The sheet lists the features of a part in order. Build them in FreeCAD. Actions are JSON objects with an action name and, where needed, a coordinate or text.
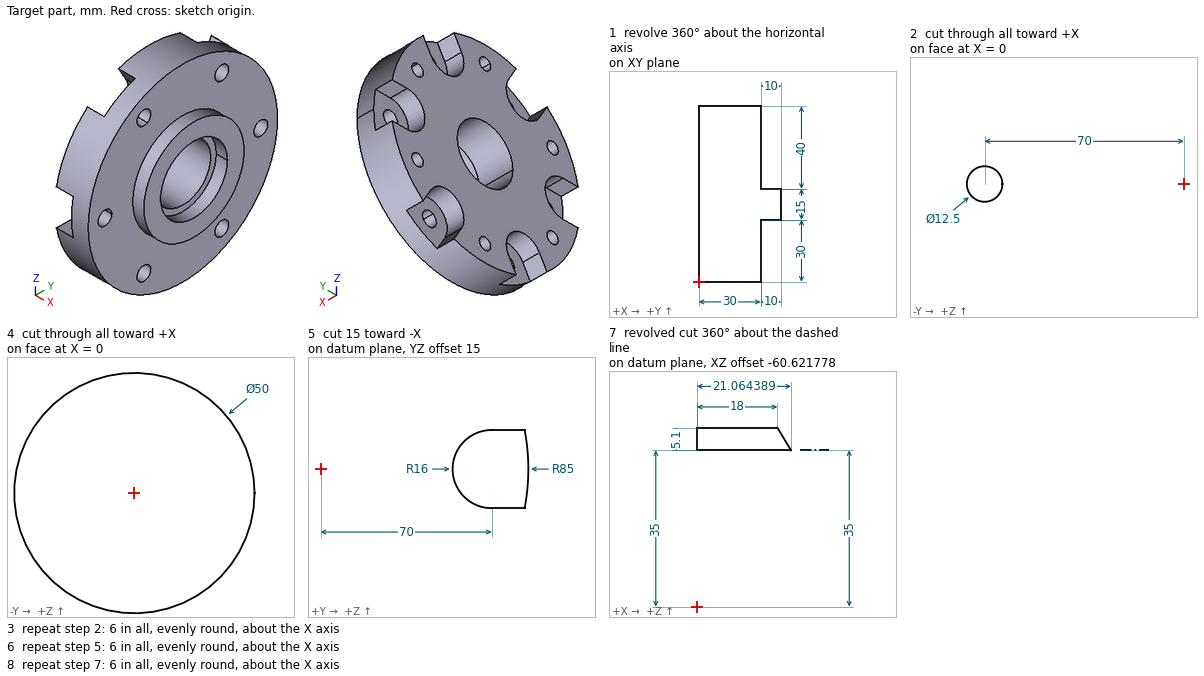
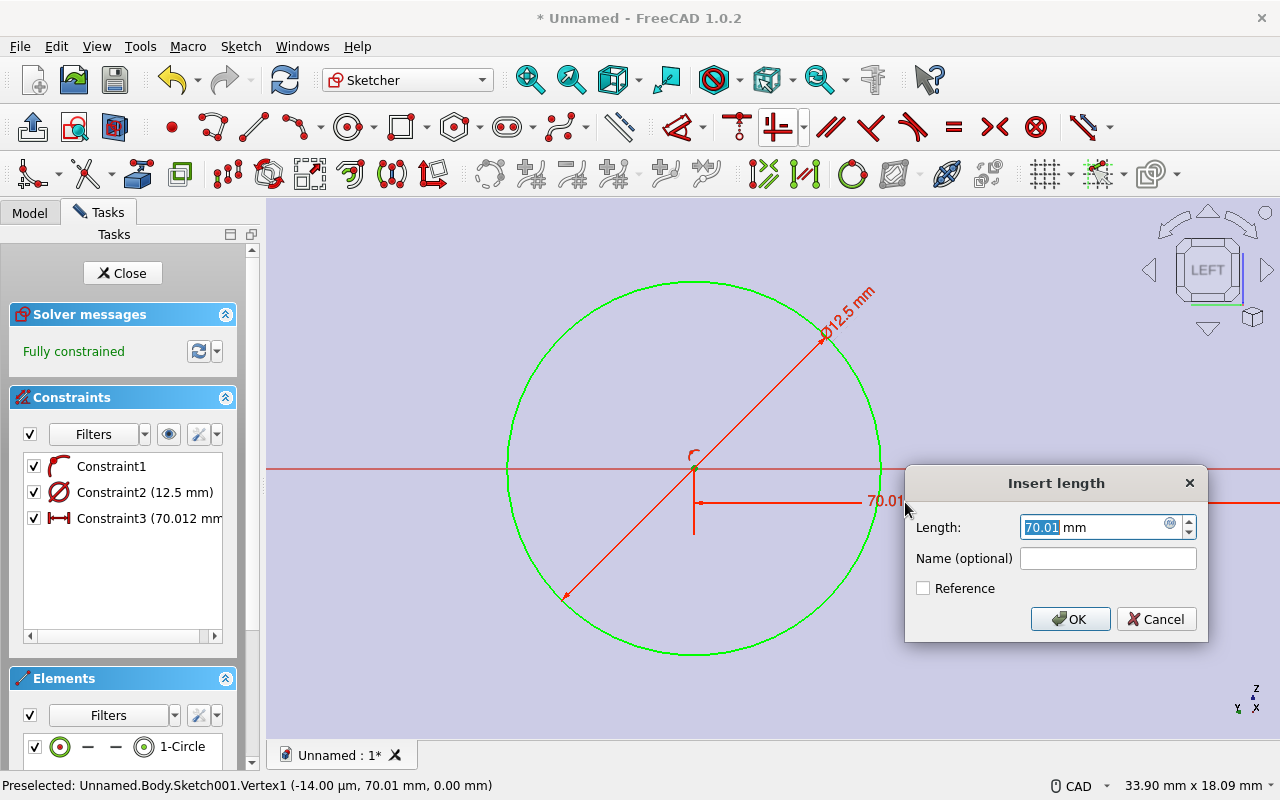
{"action": "type", "text": "70"}
{"action": "key", "text": "Return"}
{"action": "key", "text": "Escape"}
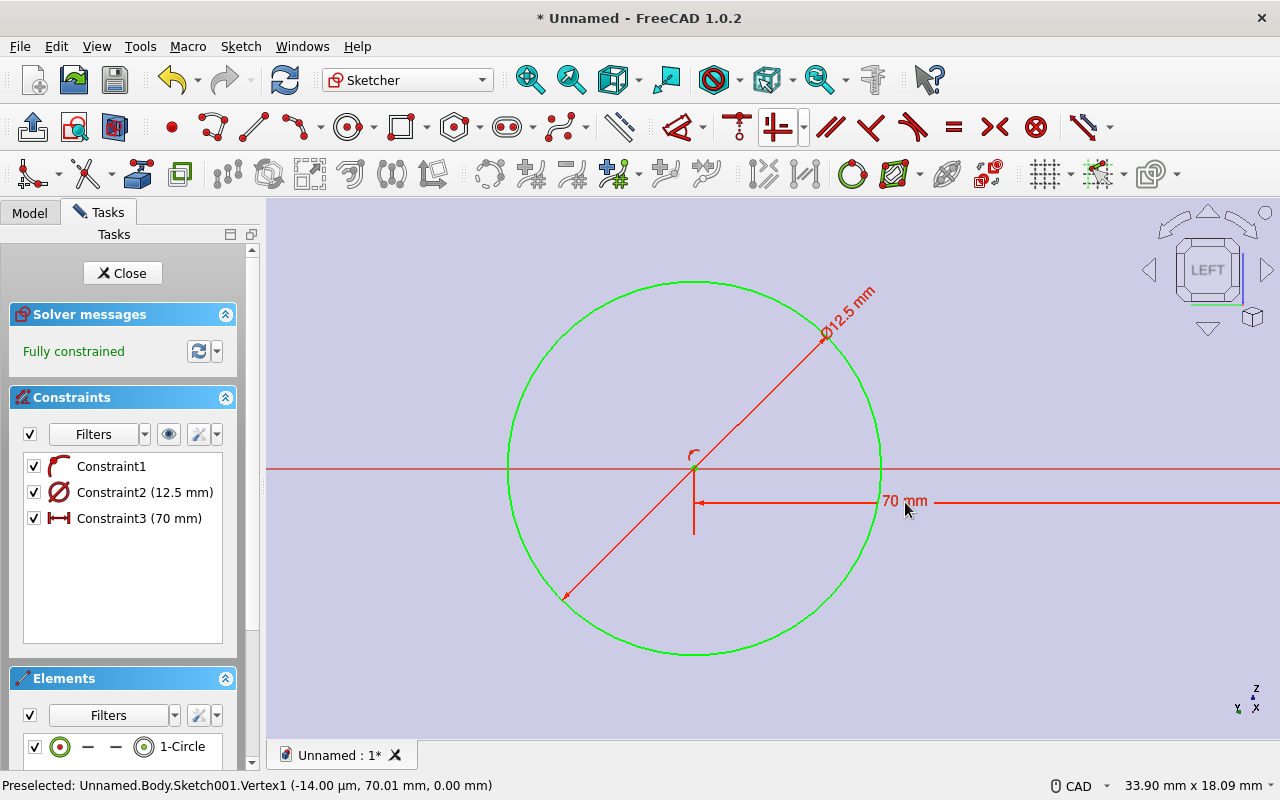
{"action": "left_click", "coordinate": [123, 273]}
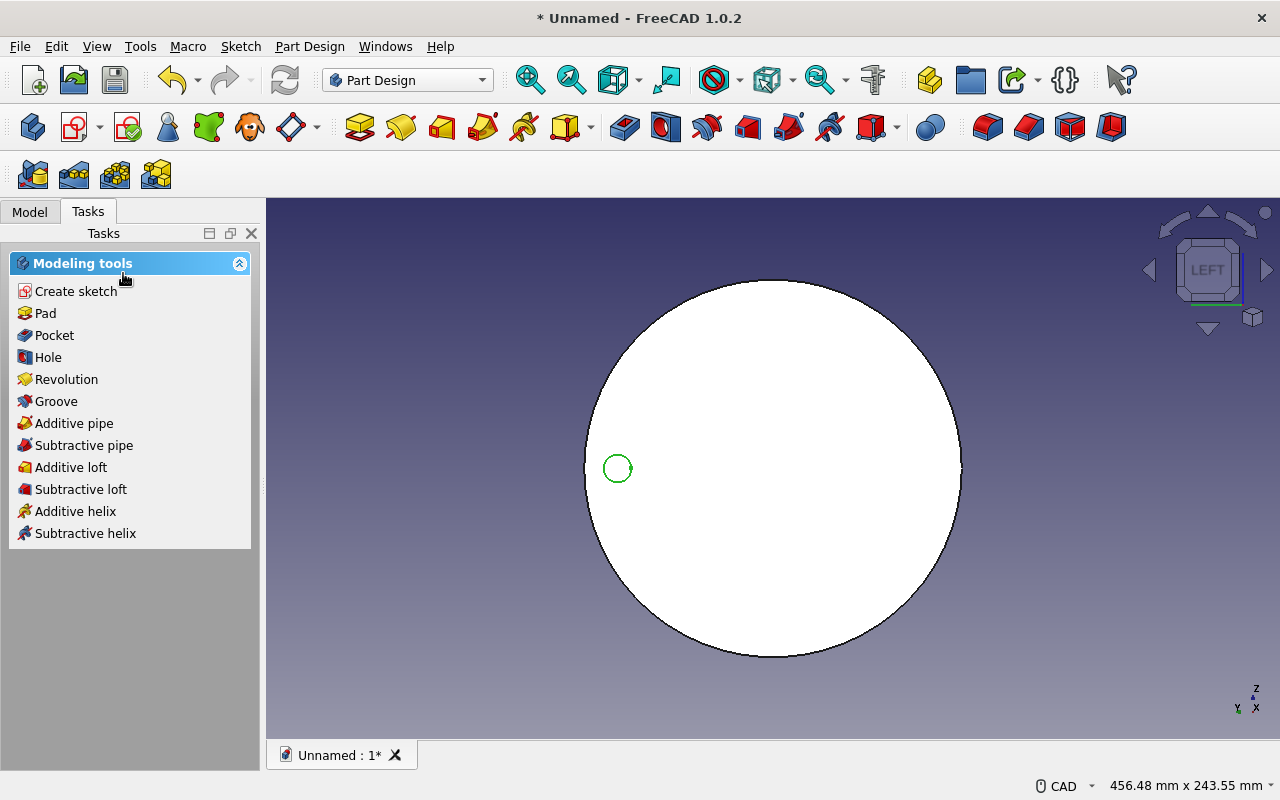
{"action": "left_click", "coordinate": [625, 128]}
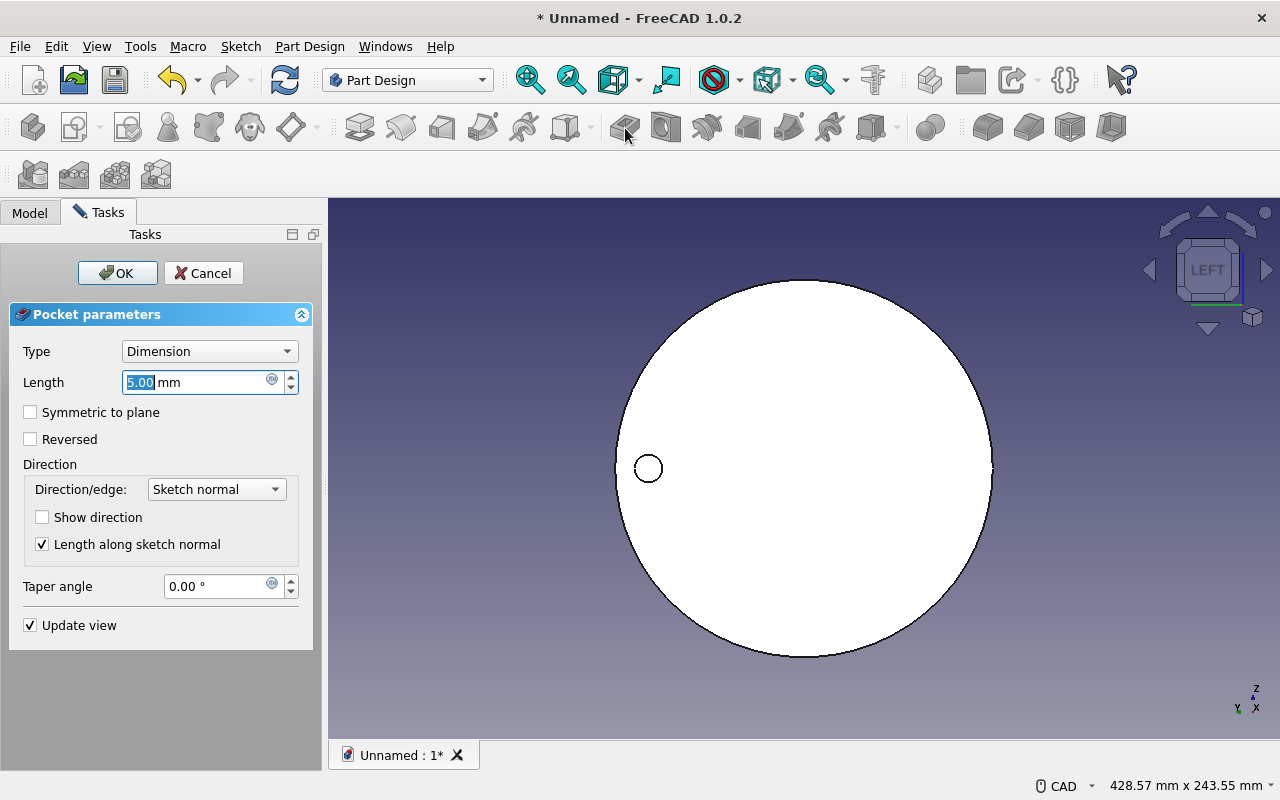
{"action": "left_click", "coordinate": [210, 352]}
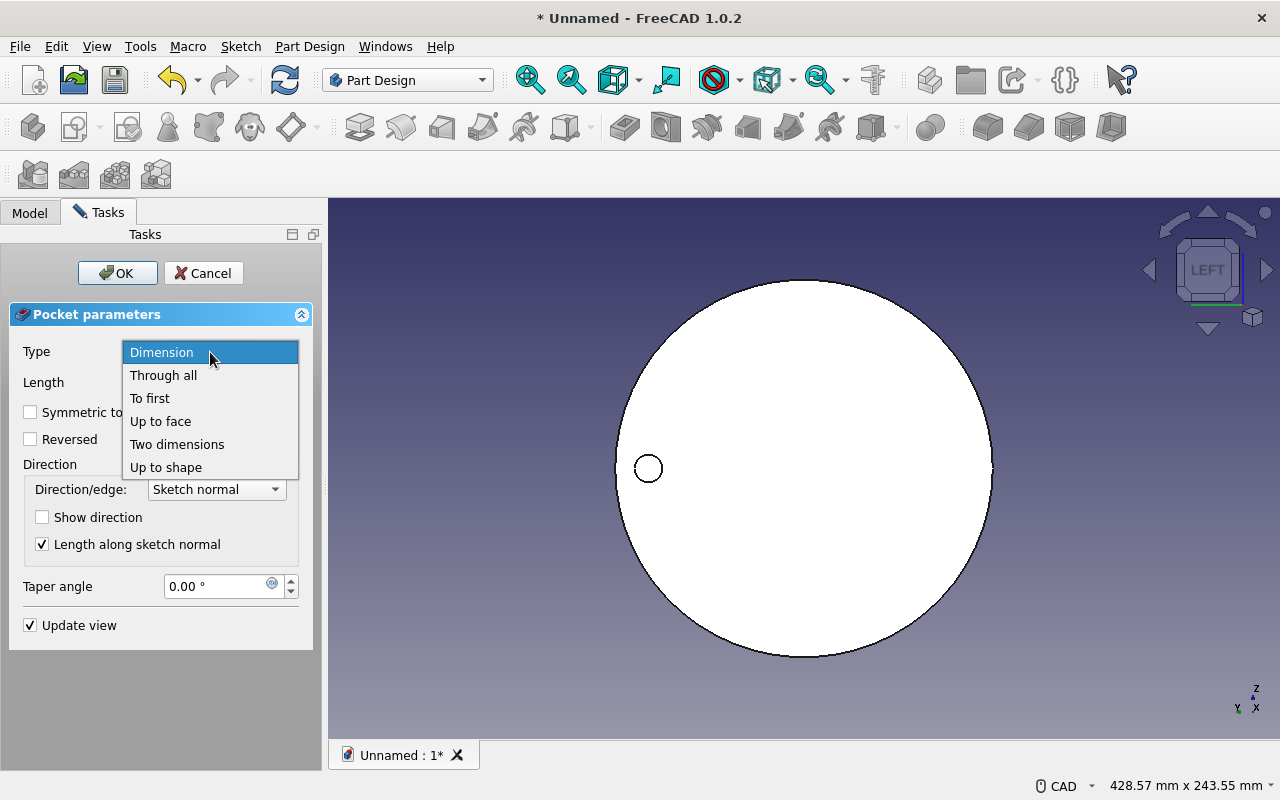
{"action": "left_click", "coordinate": [208, 376]}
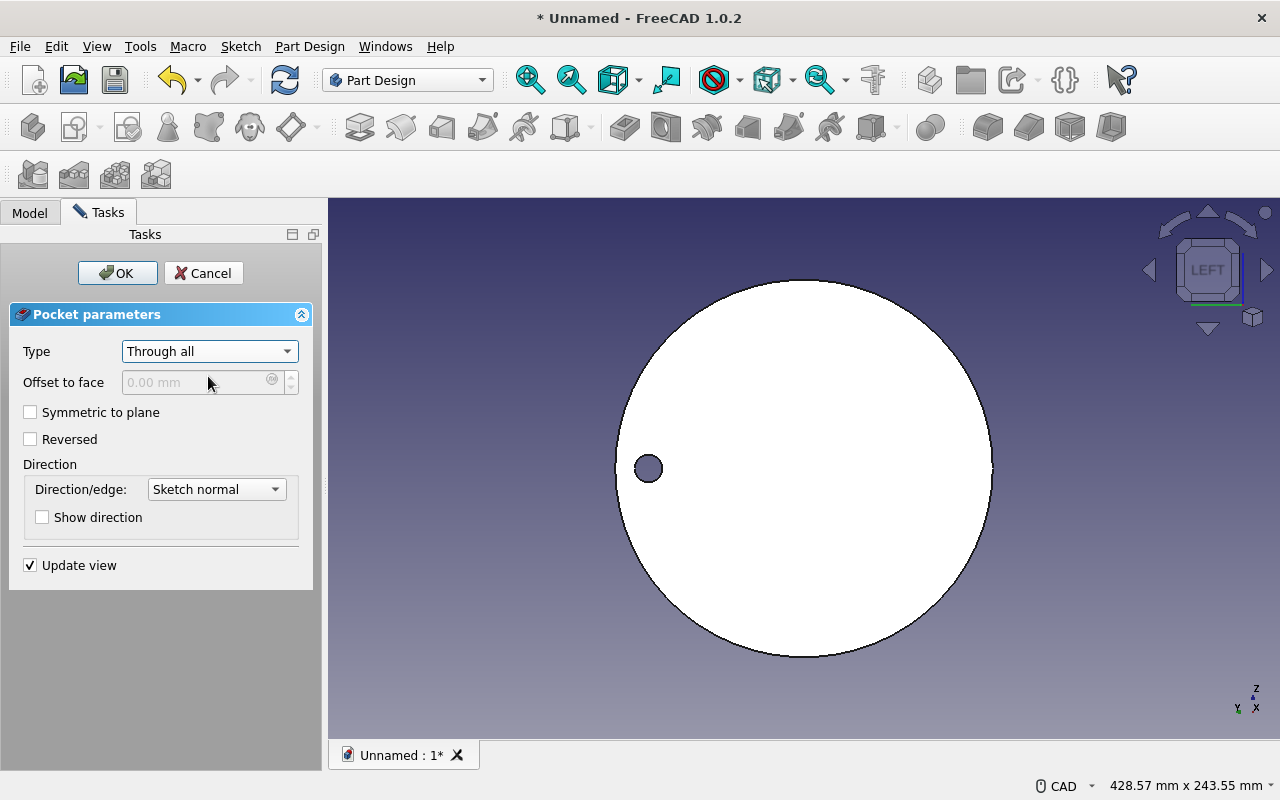
{"action": "left_click", "coordinate": [118, 273]}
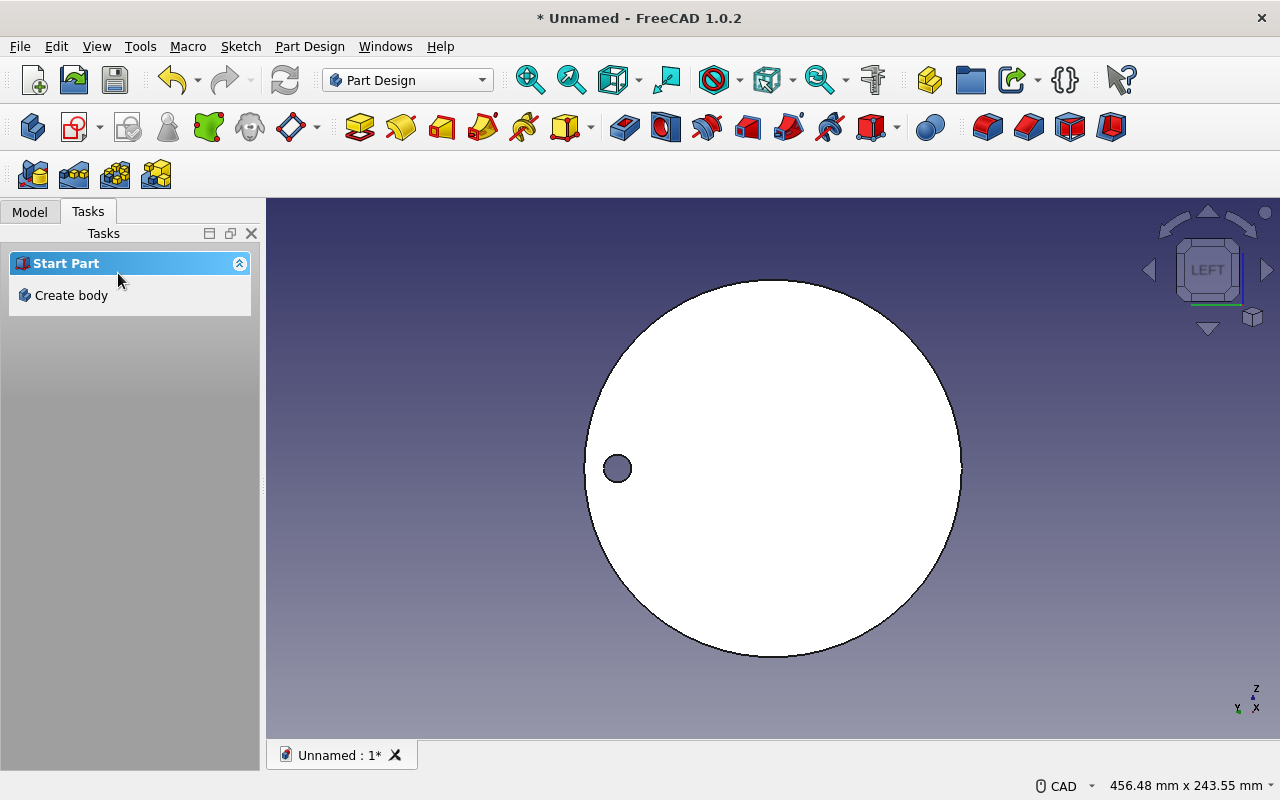
{"action": "left_click", "coordinate": [30, 212]}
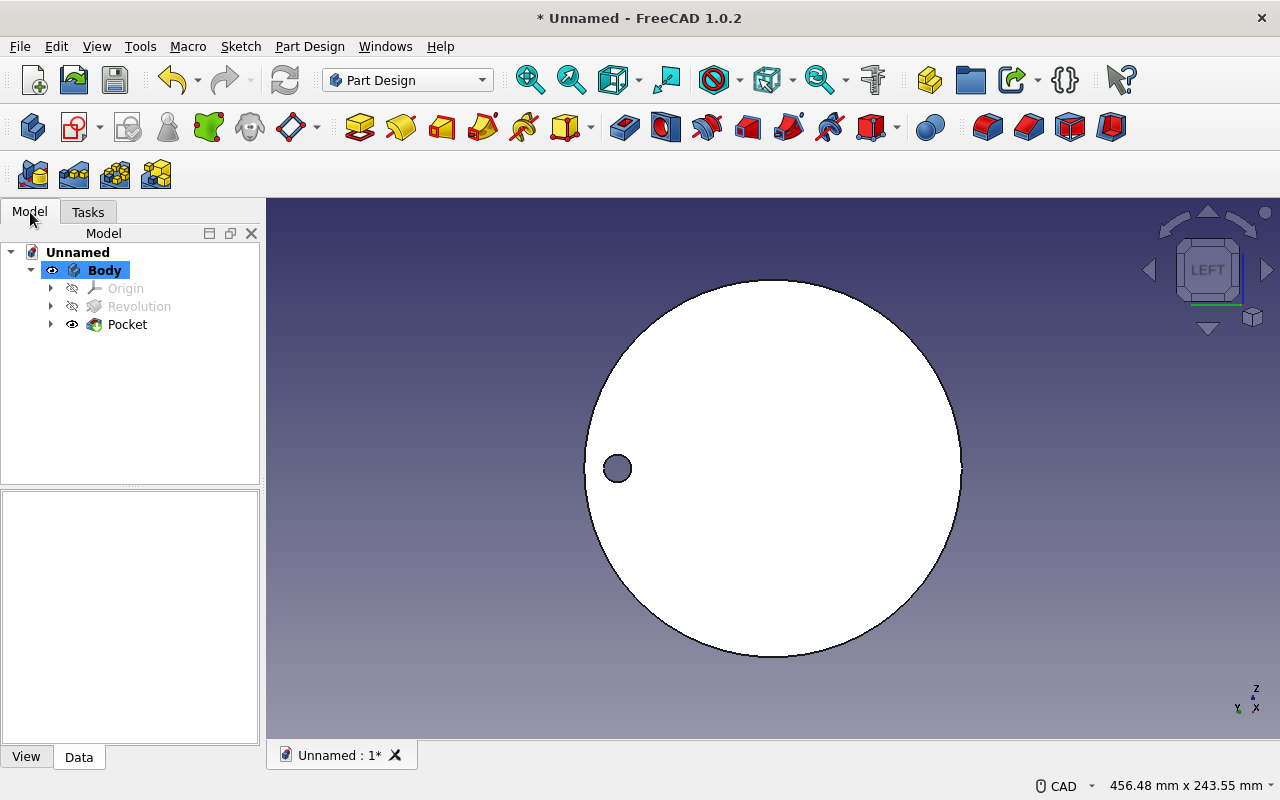
{"action": "left_click", "coordinate": [117, 324]}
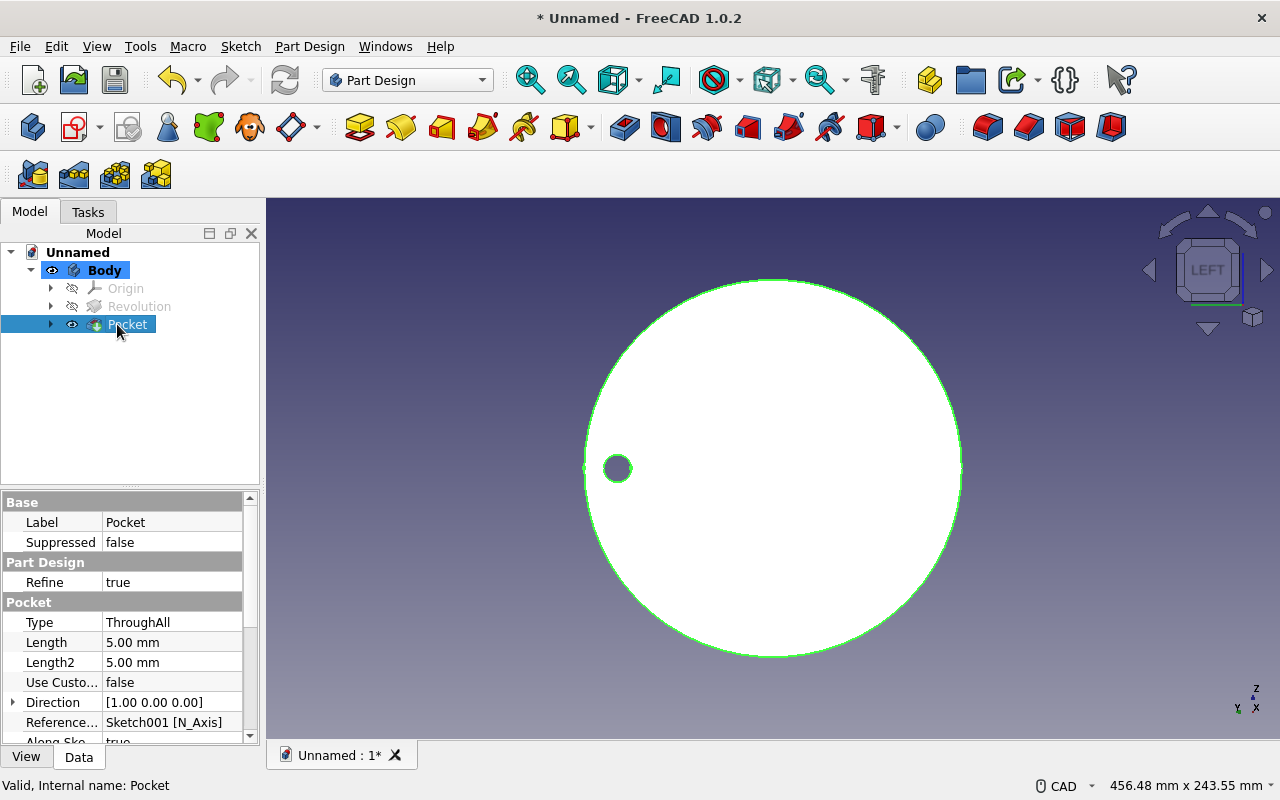
{"action": "left_click", "coordinate": [115, 174]}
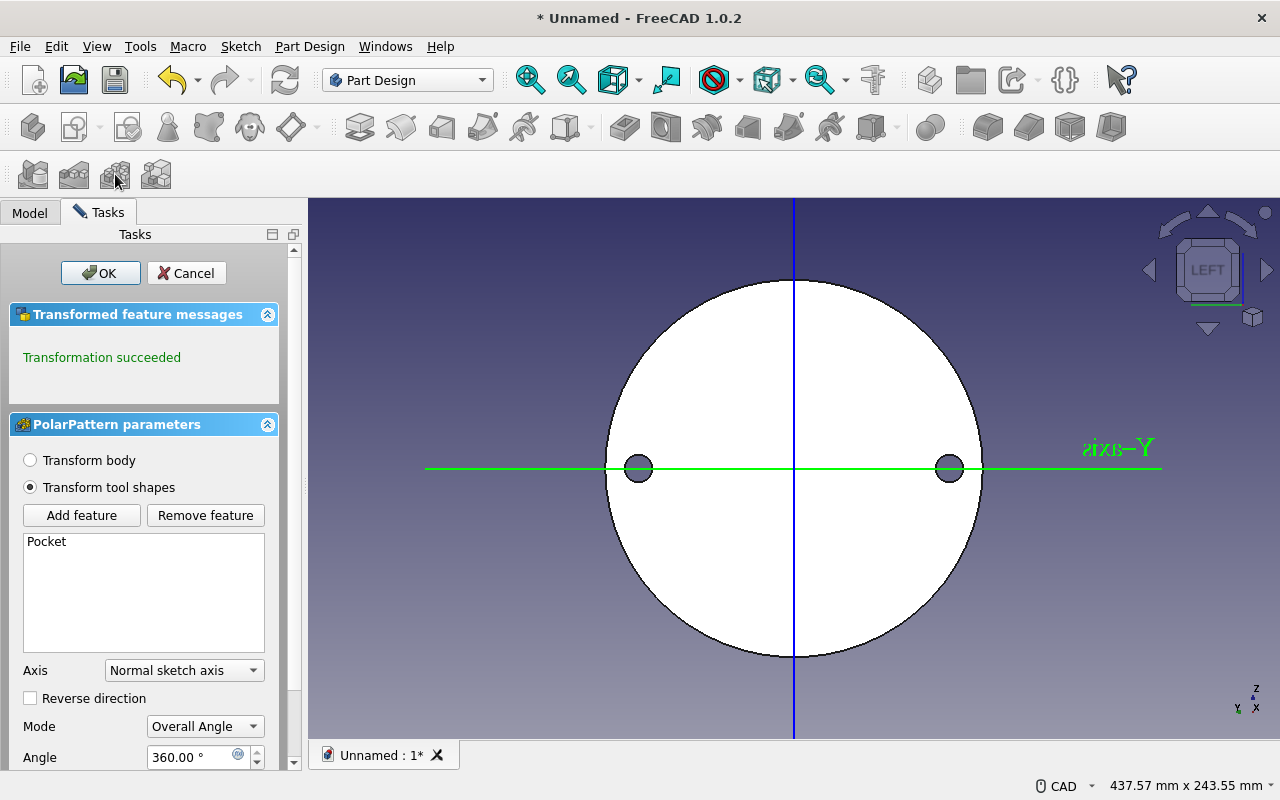
{"action": "left_click", "coordinate": [185, 670]}